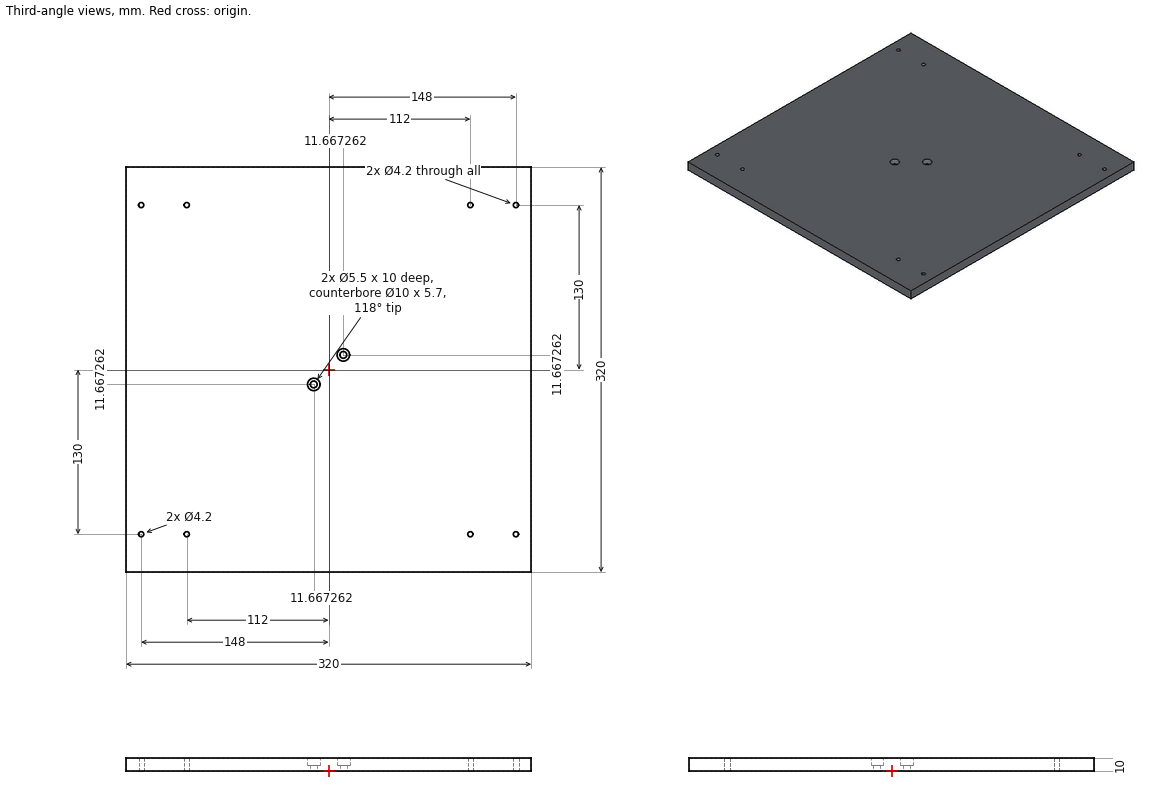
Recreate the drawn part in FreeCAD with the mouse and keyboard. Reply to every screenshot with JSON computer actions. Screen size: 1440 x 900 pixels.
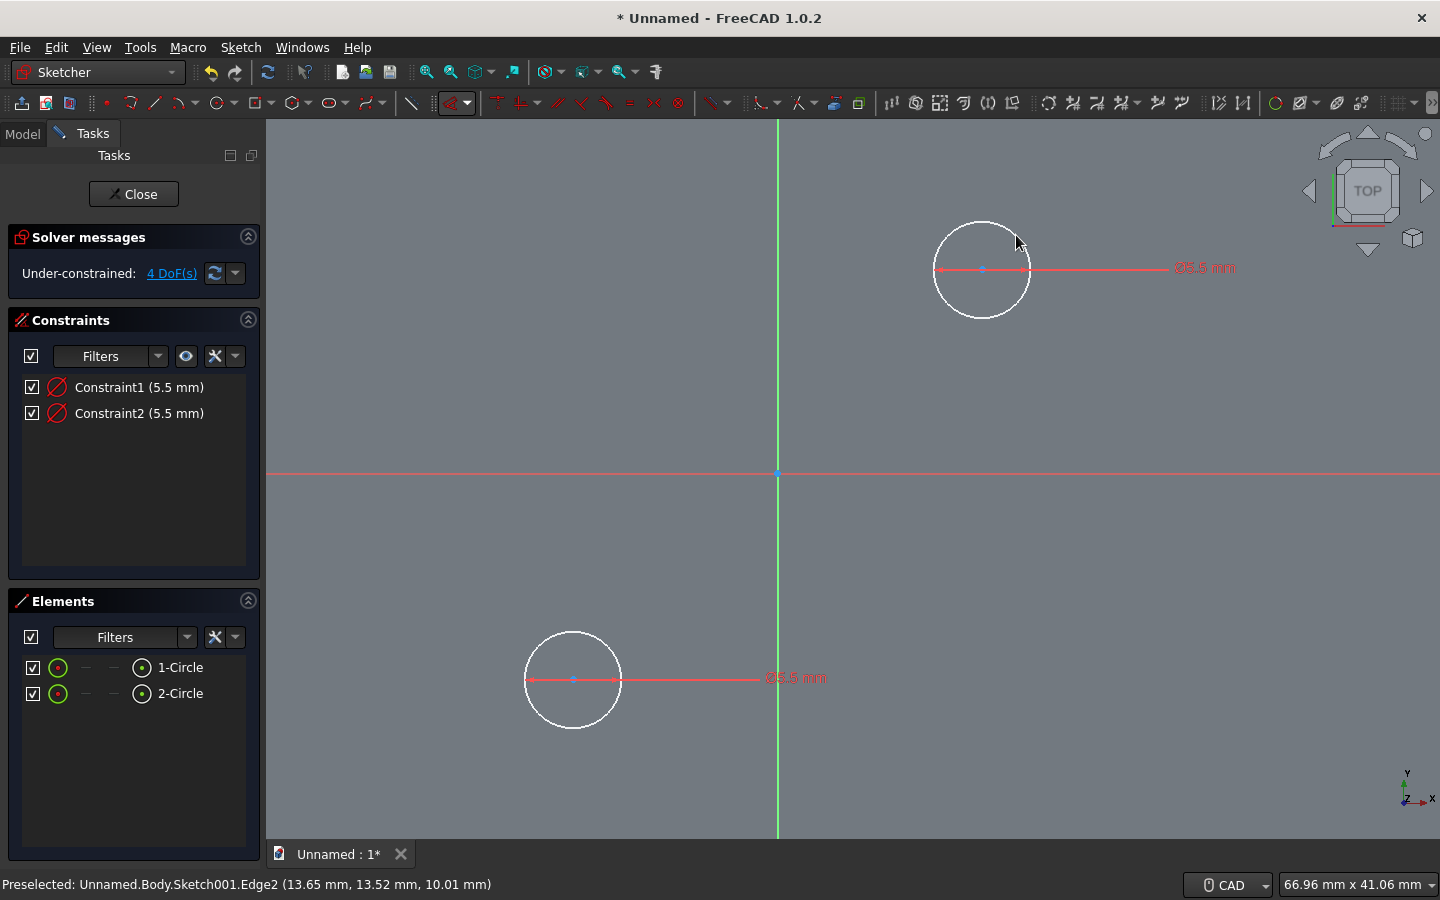
{"action": "key", "text": "d"}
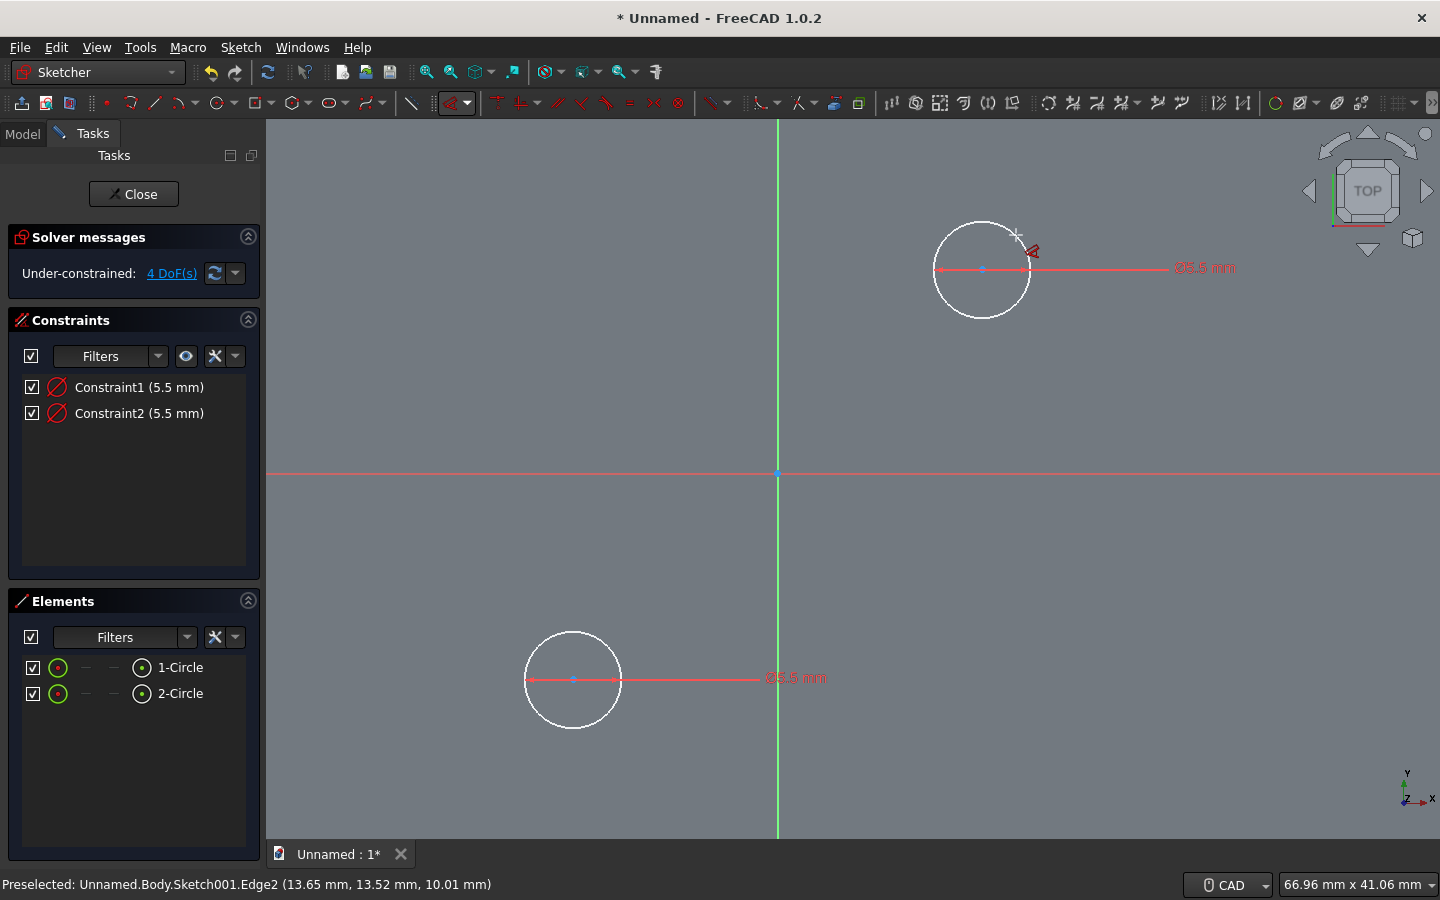
{"action": "left_click", "coordinate": [573, 680]}
{"action": "left_click", "coordinate": [675, 714]}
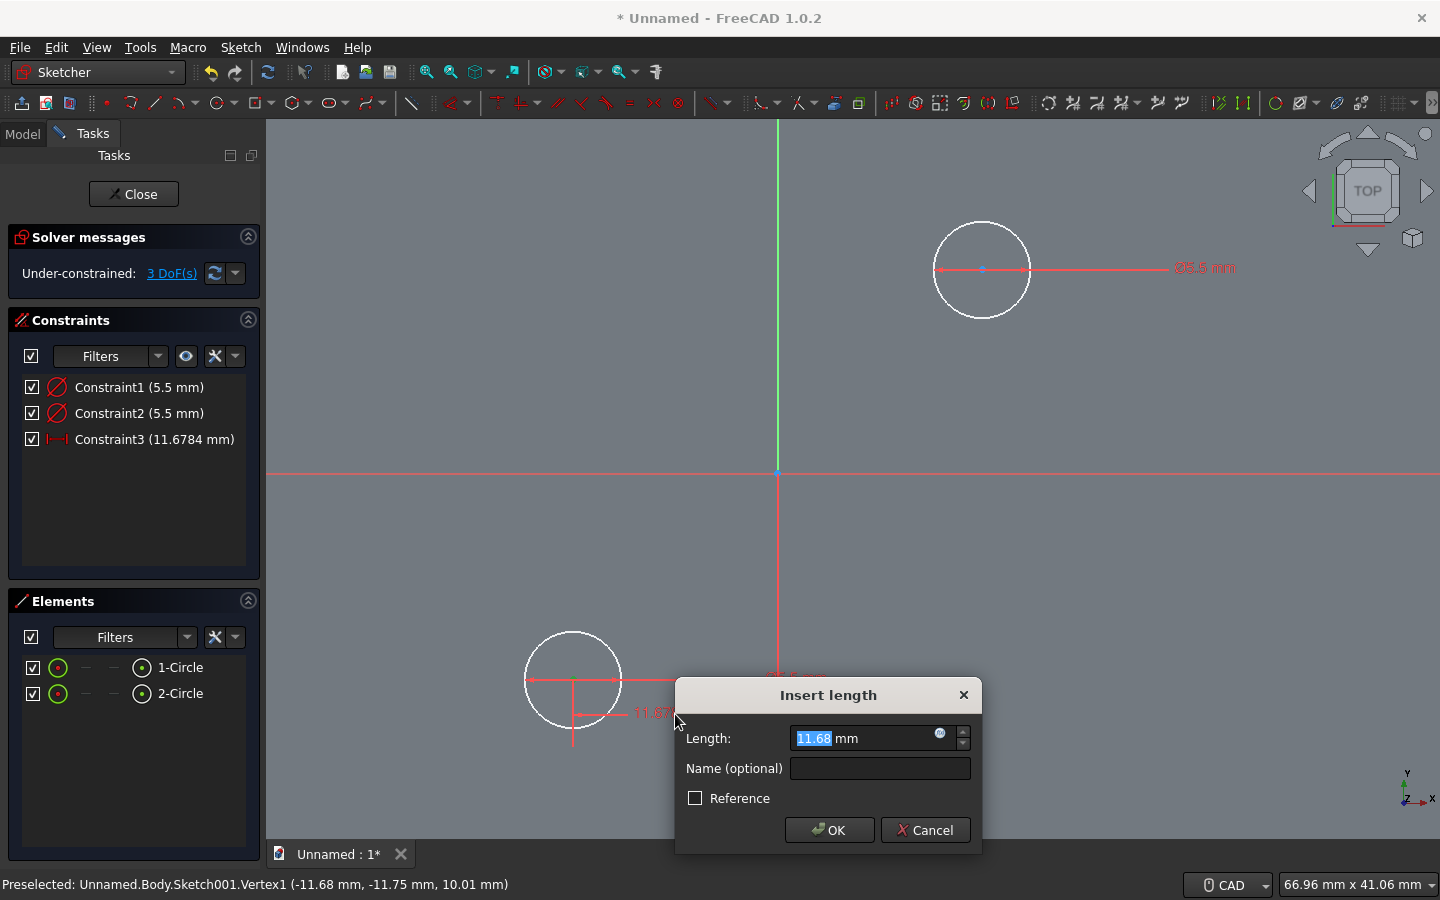
{"action": "type", "text": "11.667262"}
{"action": "key", "text": "Return"}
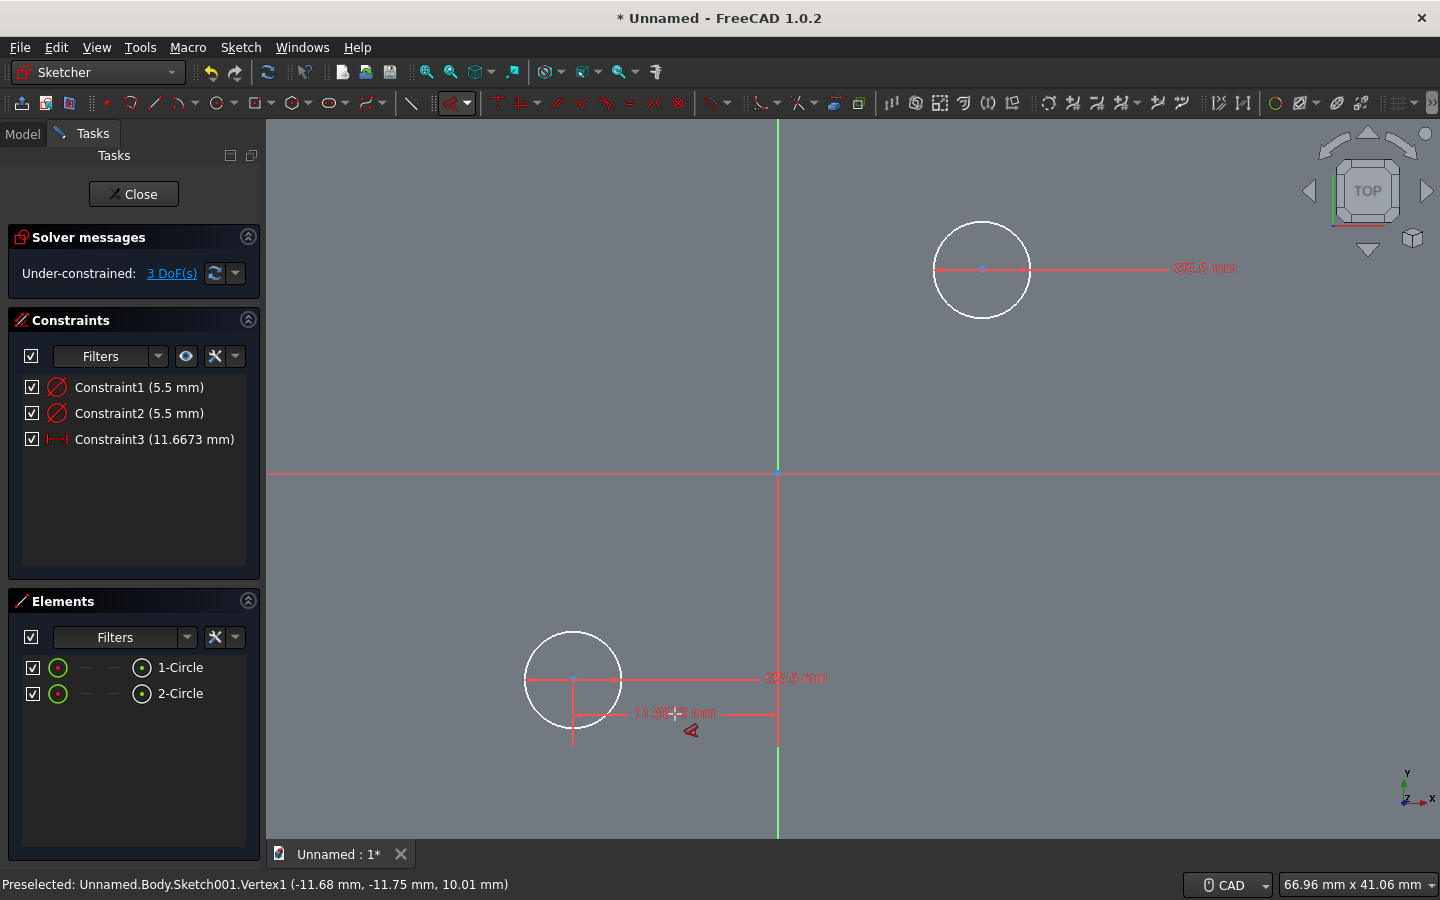
{"action": "left_click", "coordinate": [573, 680]}
{"action": "left_click", "coordinate": [539, 577]}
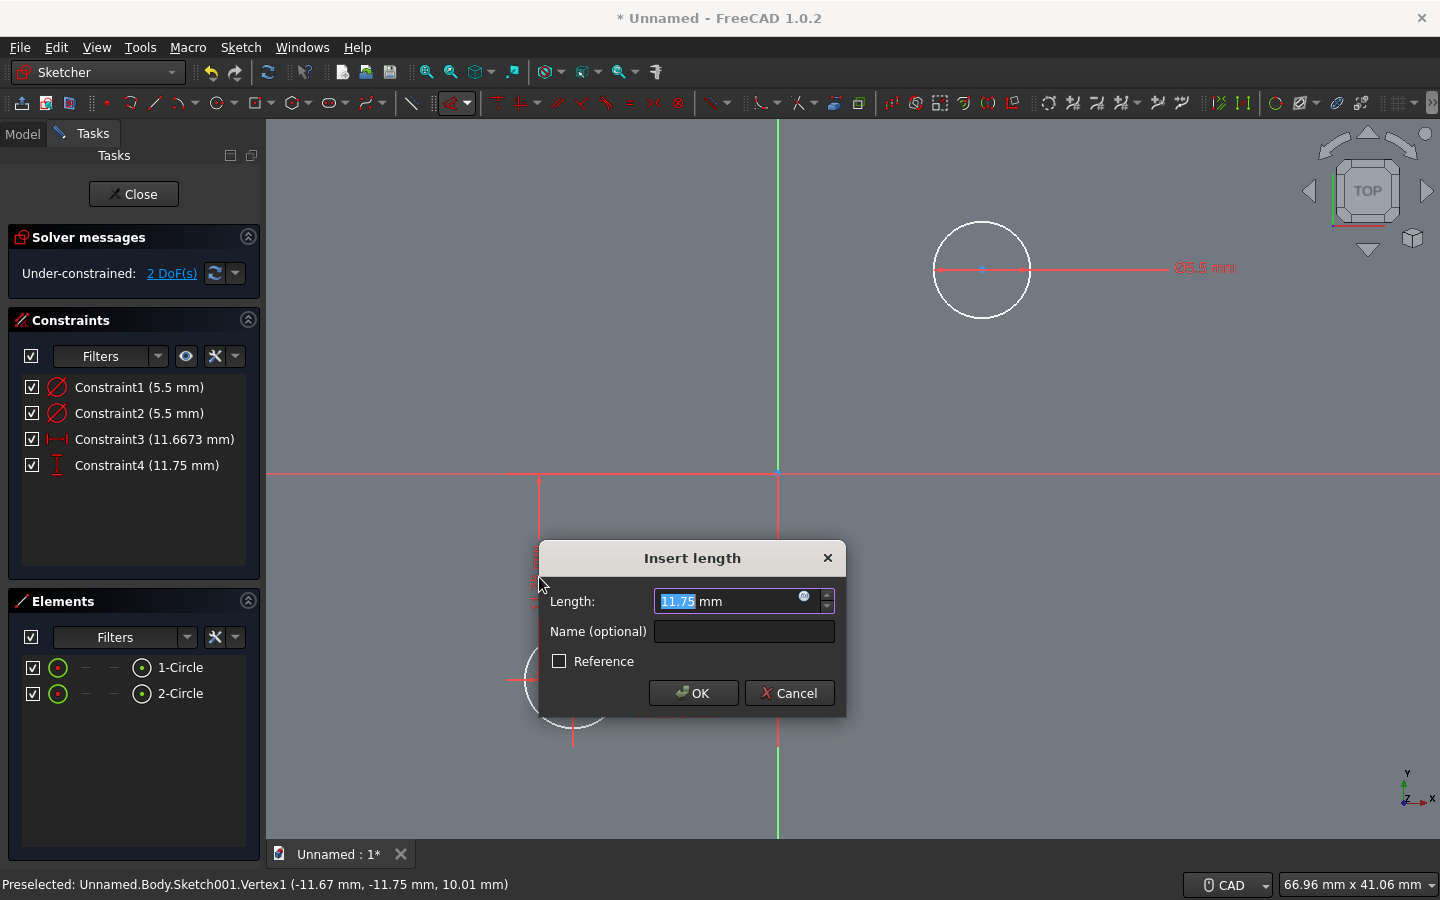
{"action": "type", "text": "11.667262"}
{"action": "key", "text": "Return"}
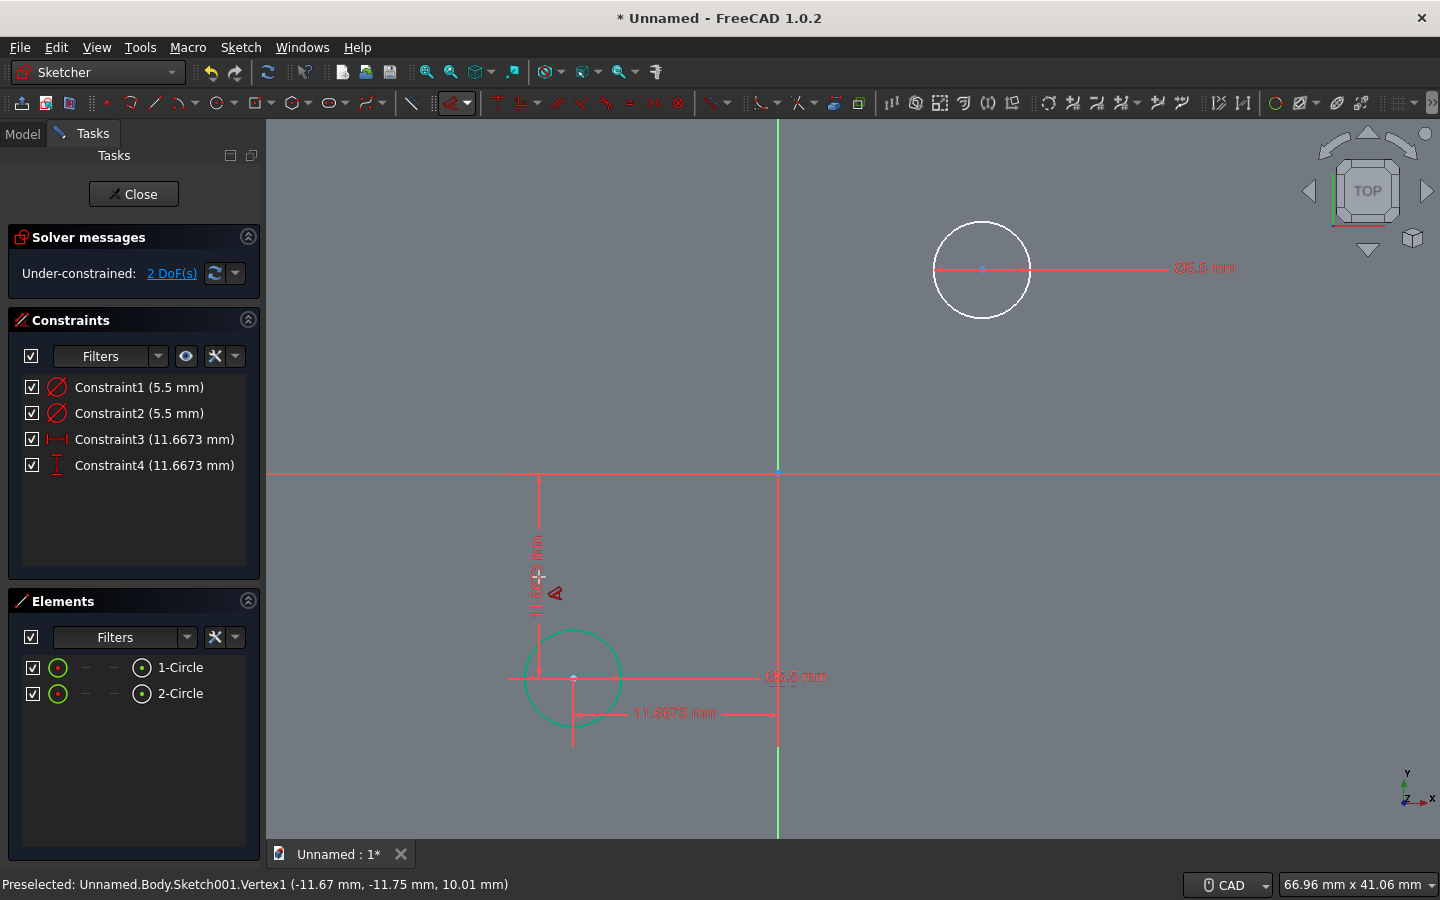
{"action": "left_click", "coordinate": [982, 270]}
{"action": "left_click", "coordinate": [880, 236]}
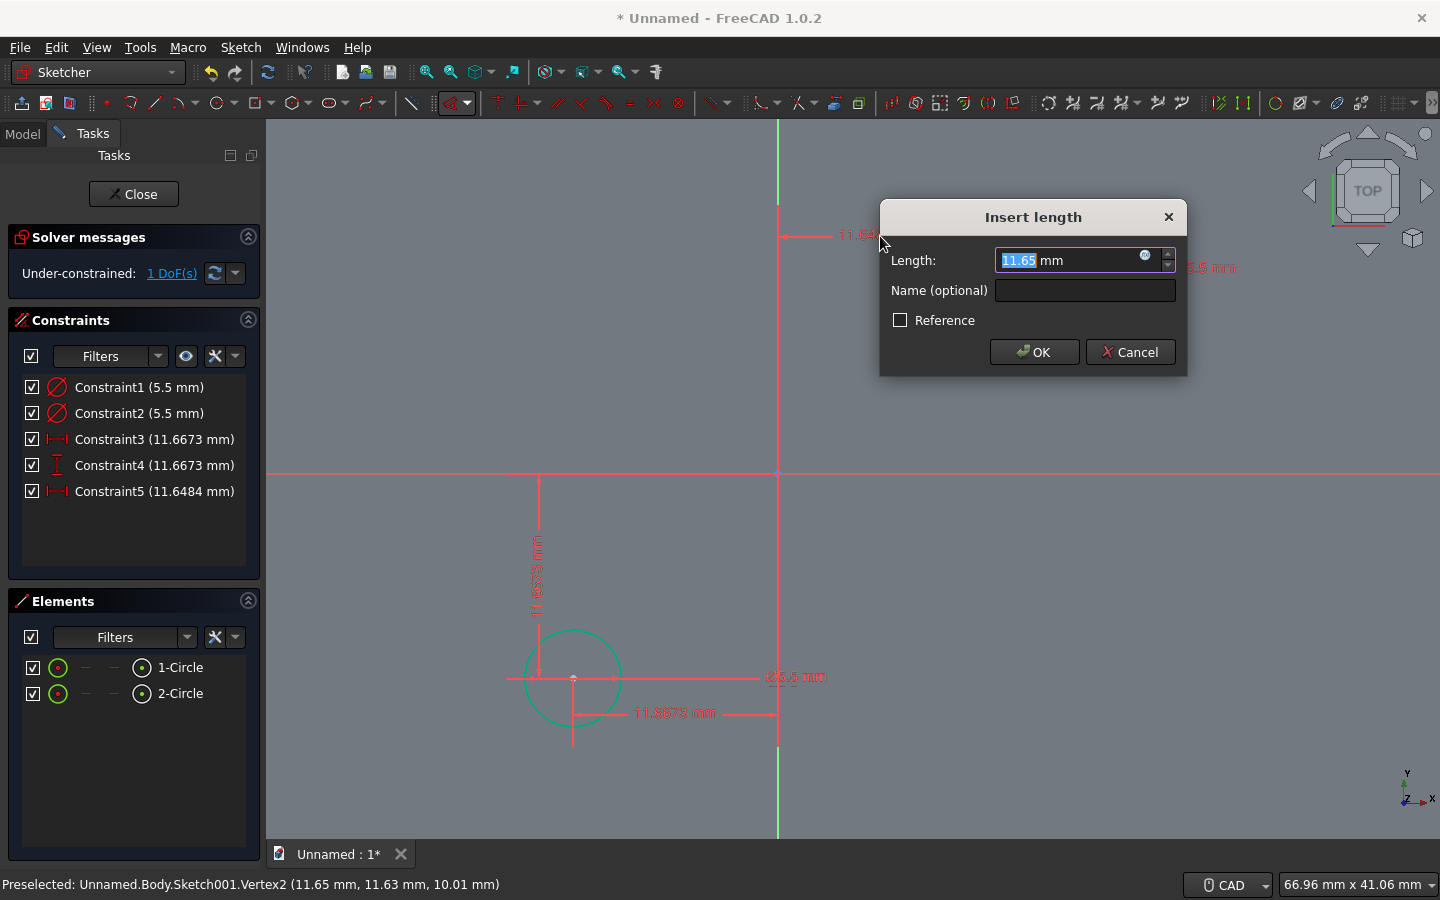
{"action": "type", "text": "11.667262"}
{"action": "key", "text": "Return"}